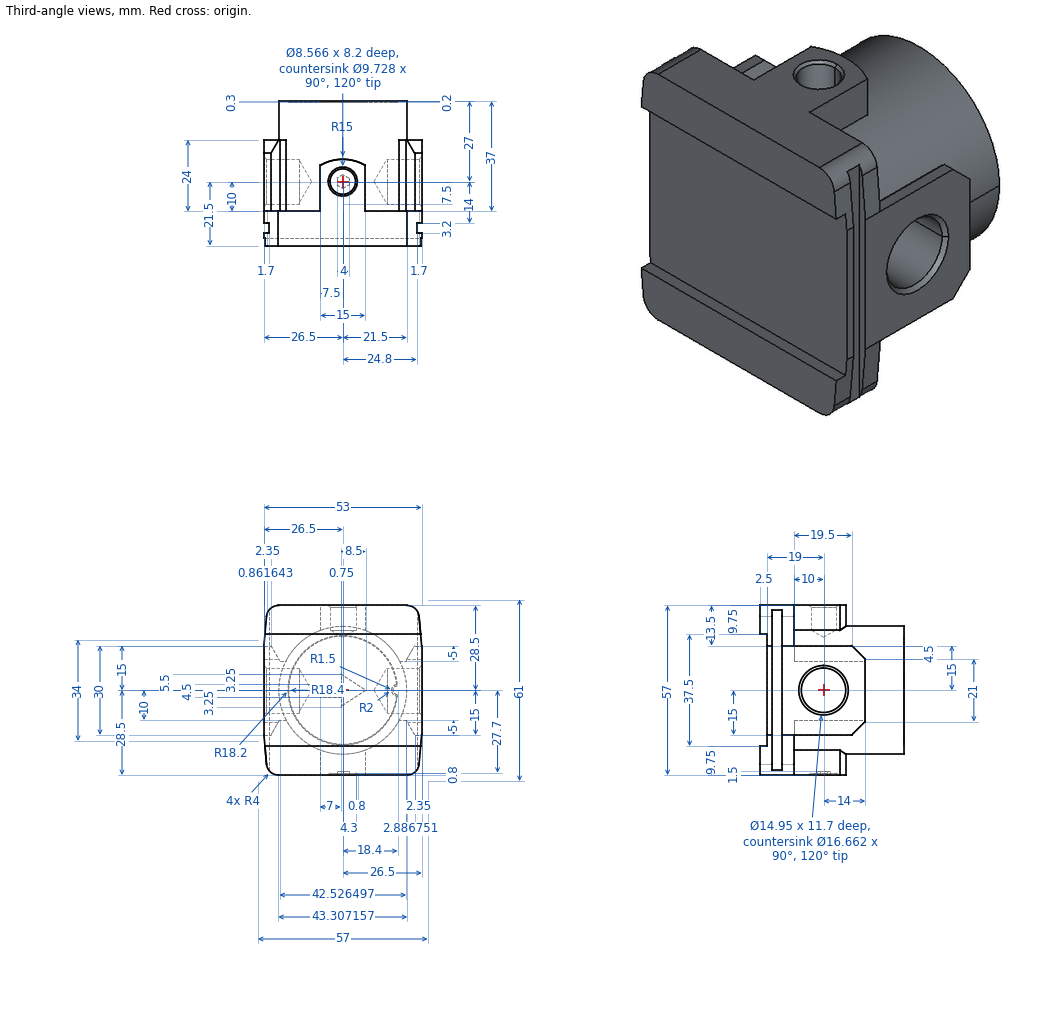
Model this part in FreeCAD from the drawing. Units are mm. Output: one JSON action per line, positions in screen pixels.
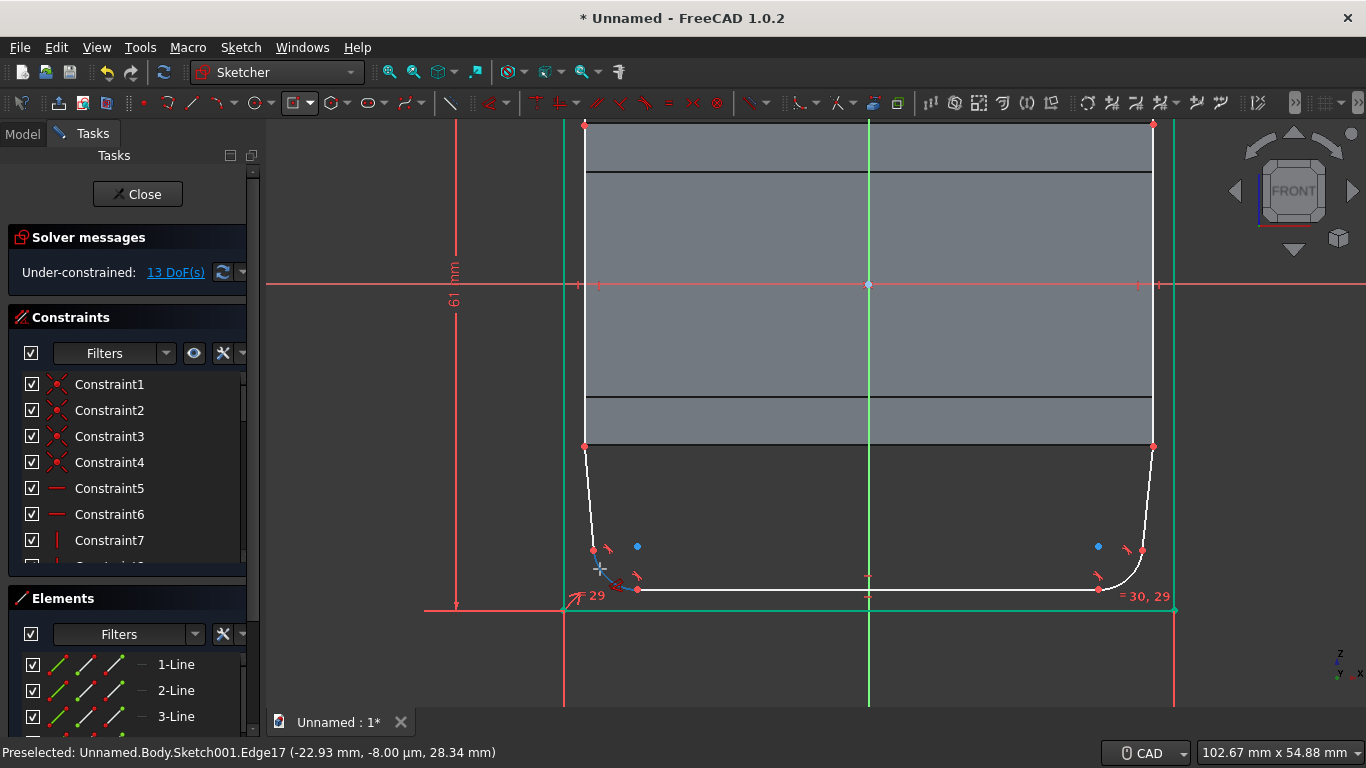
{"action": "left_click", "coordinate": [600, 568]}
{"action": "left_click", "coordinate": [702, 508]}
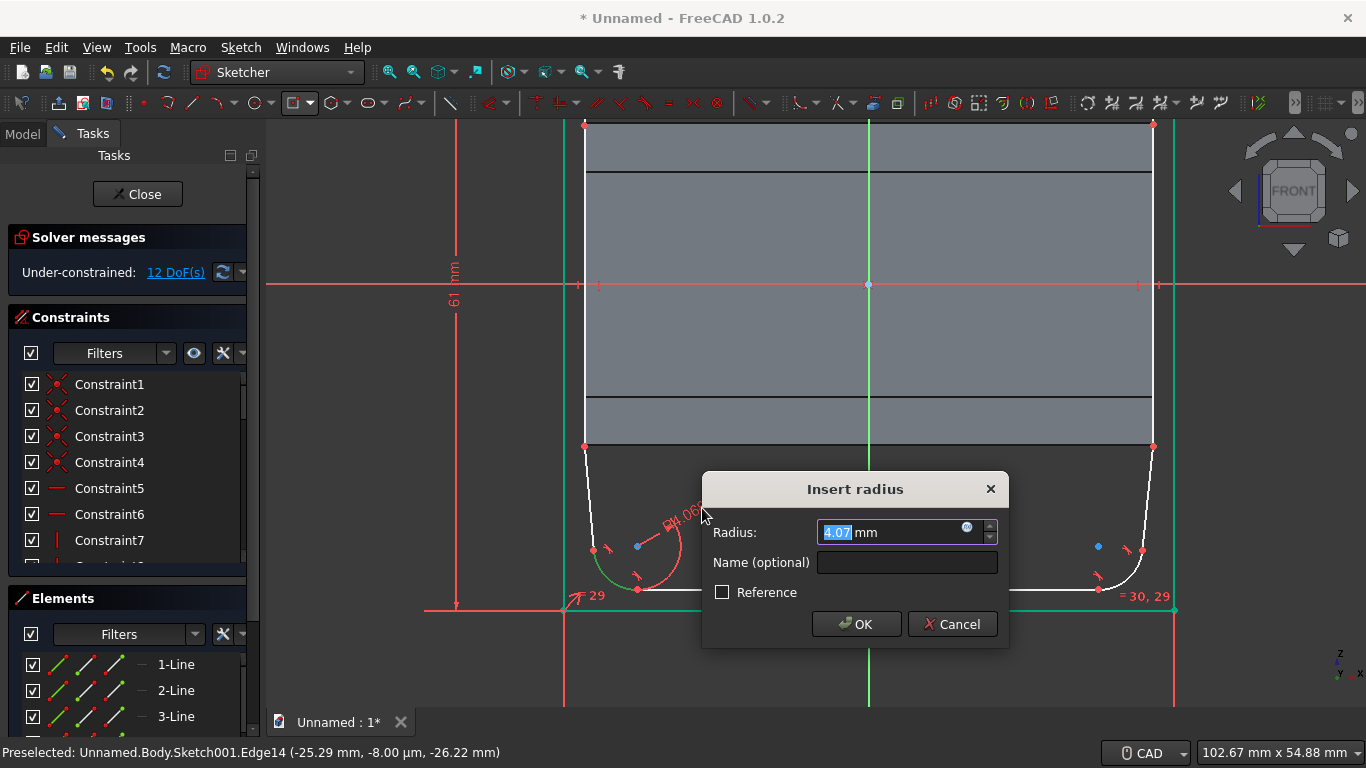
{"action": "type", "text": "4"}
{"action": "key", "text": "Return"}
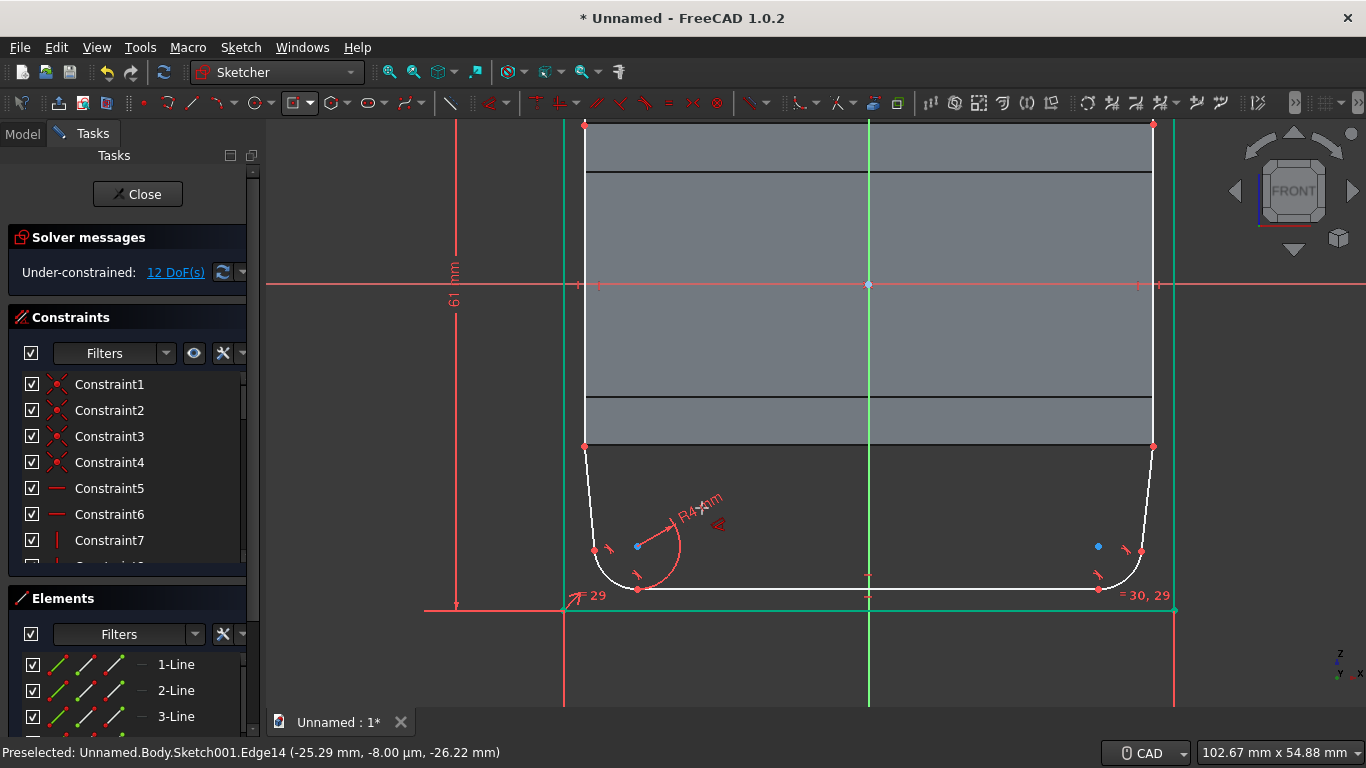
{"action": "left_click", "coordinate": [585, 222]}
{"action": "left_click", "coordinate": [619, 228]}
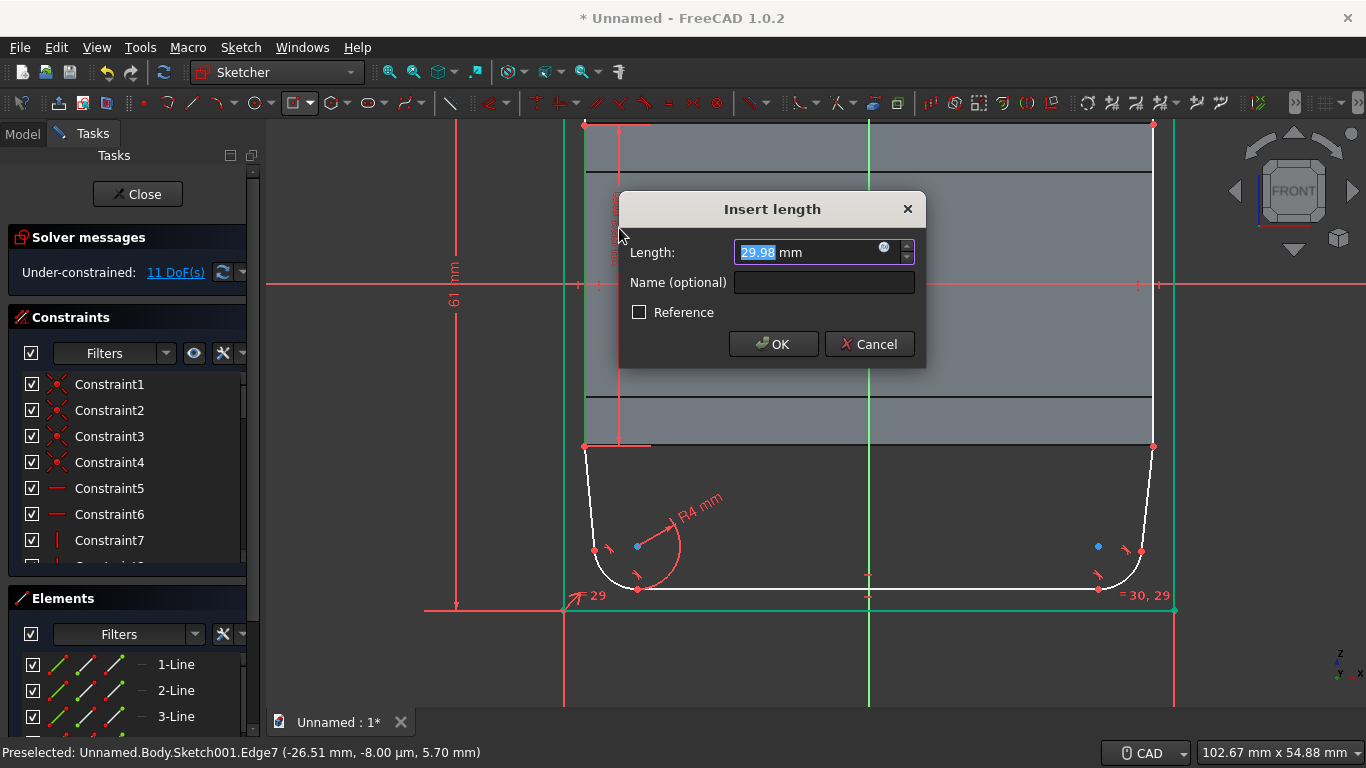
{"action": "type", "text": "30"}
{"action": "key", "text": "Return"}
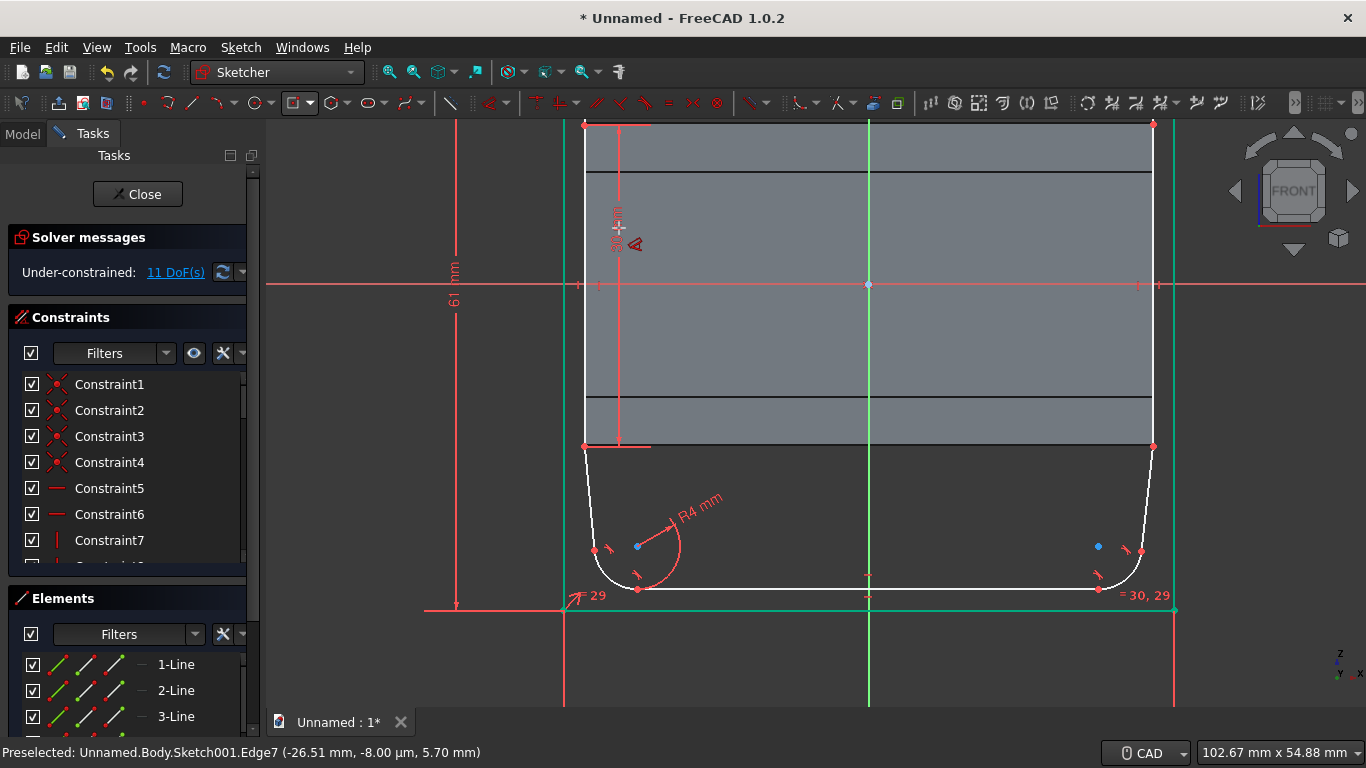
{"action": "left_click", "coordinate": [1153, 350]}
{"action": "left_click", "coordinate": [1119, 228]}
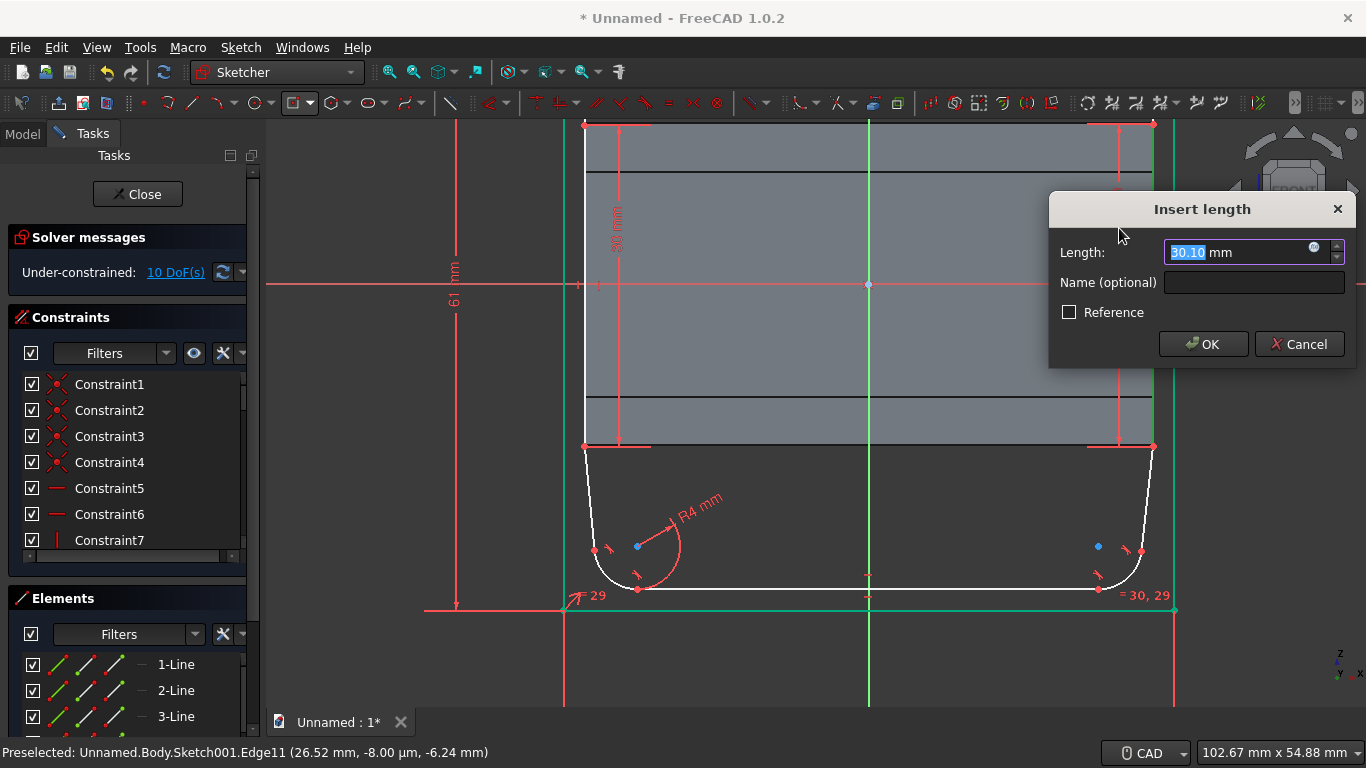
{"action": "type", "text": "30"}
{"action": "key", "text": "Return"}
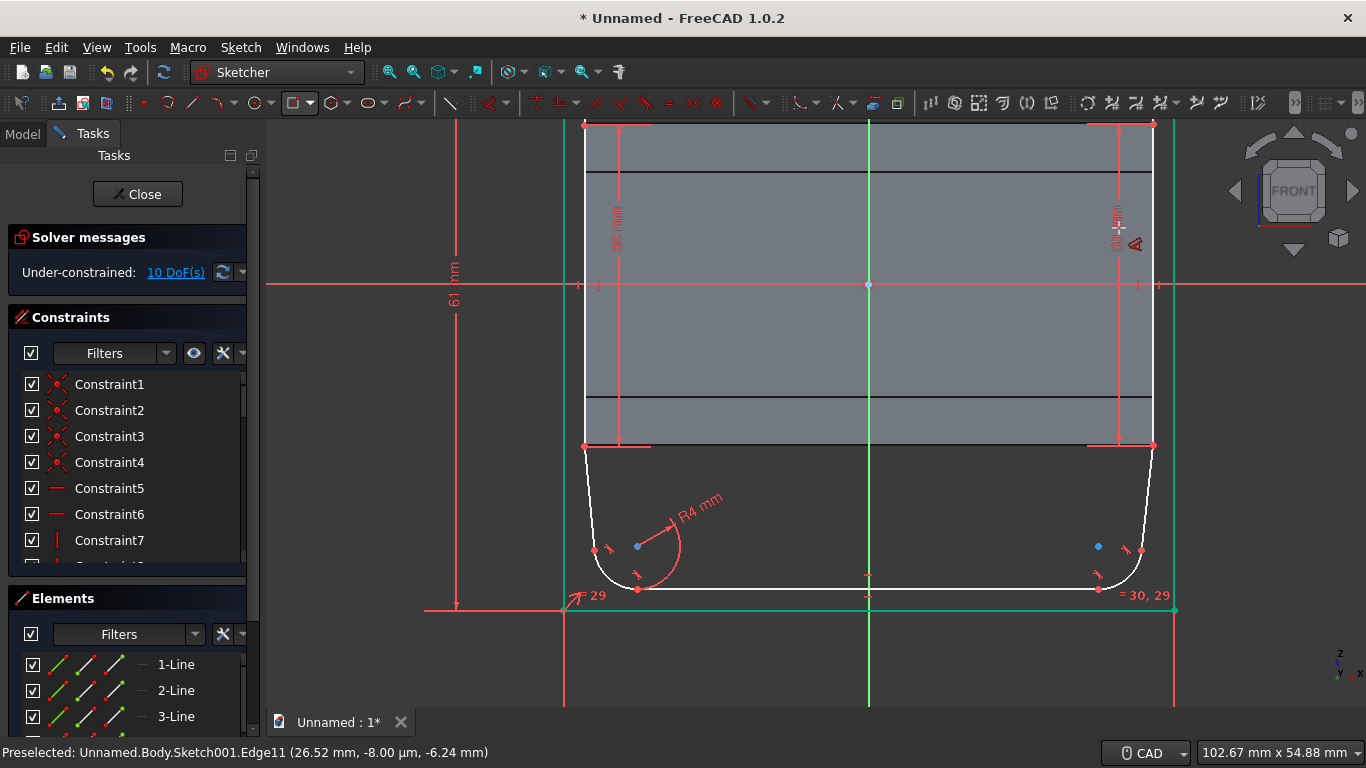
{"action": "scroll", "coordinate": [600, 570], "scroll_direction": "down", "scroll_amount": 3}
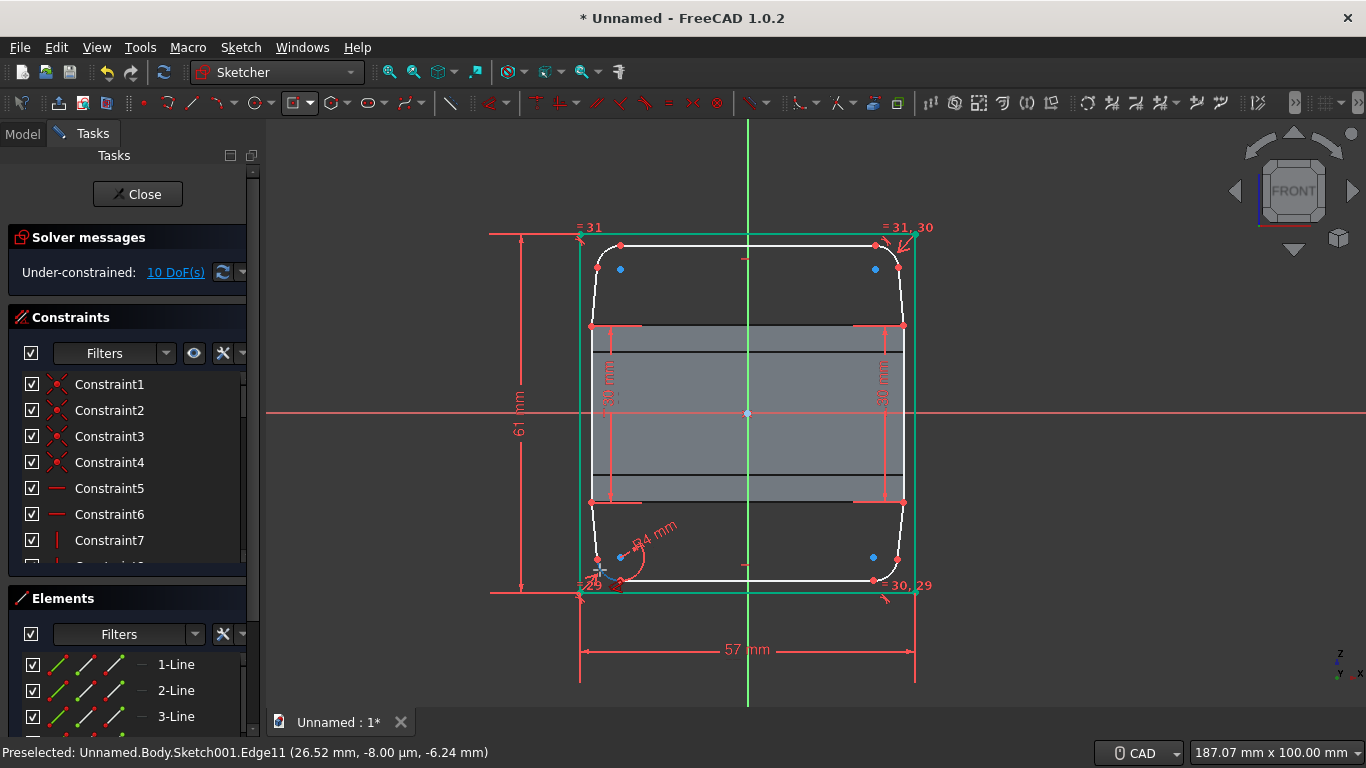
{"action": "left_click", "coordinate": [592, 326]}
{"action": "left_click", "coordinate": [558, 350]}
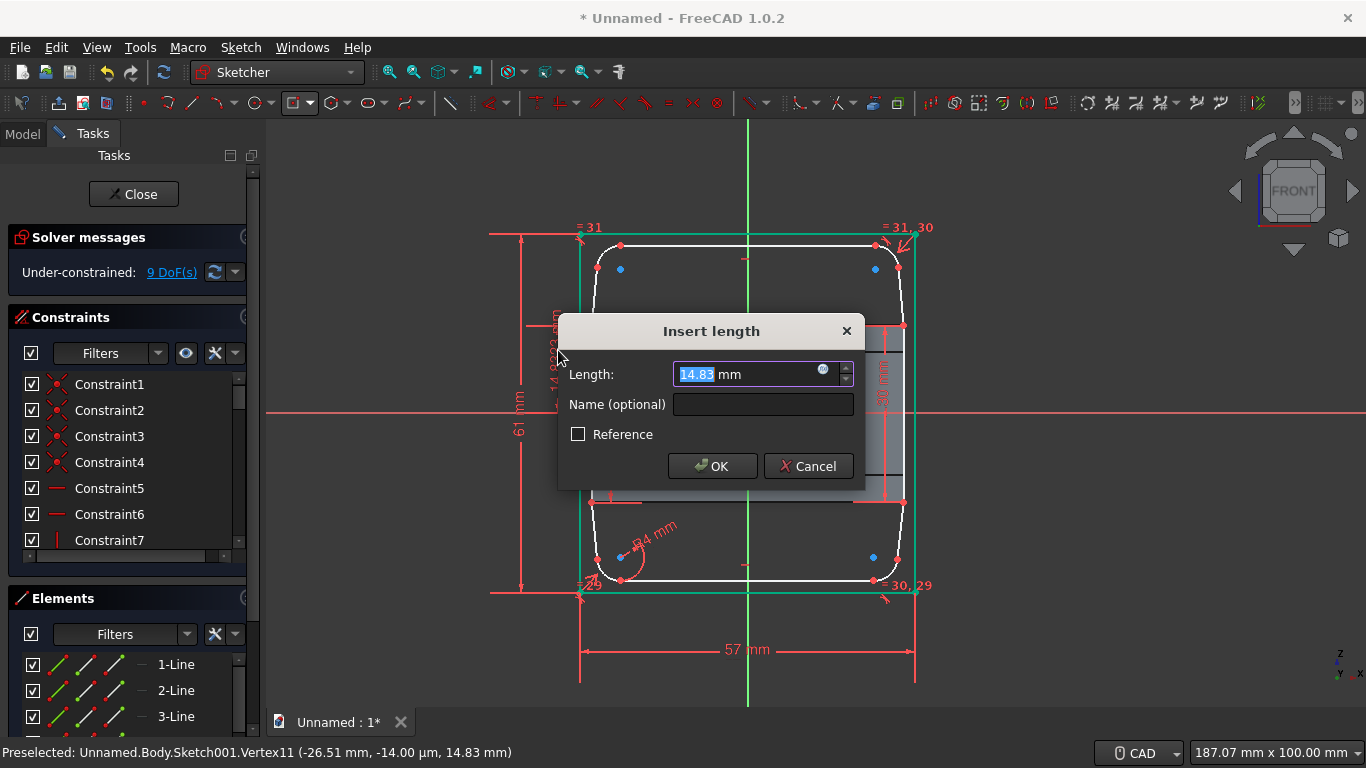
{"action": "type", "text": "15"}
{"action": "key", "text": "Return"}